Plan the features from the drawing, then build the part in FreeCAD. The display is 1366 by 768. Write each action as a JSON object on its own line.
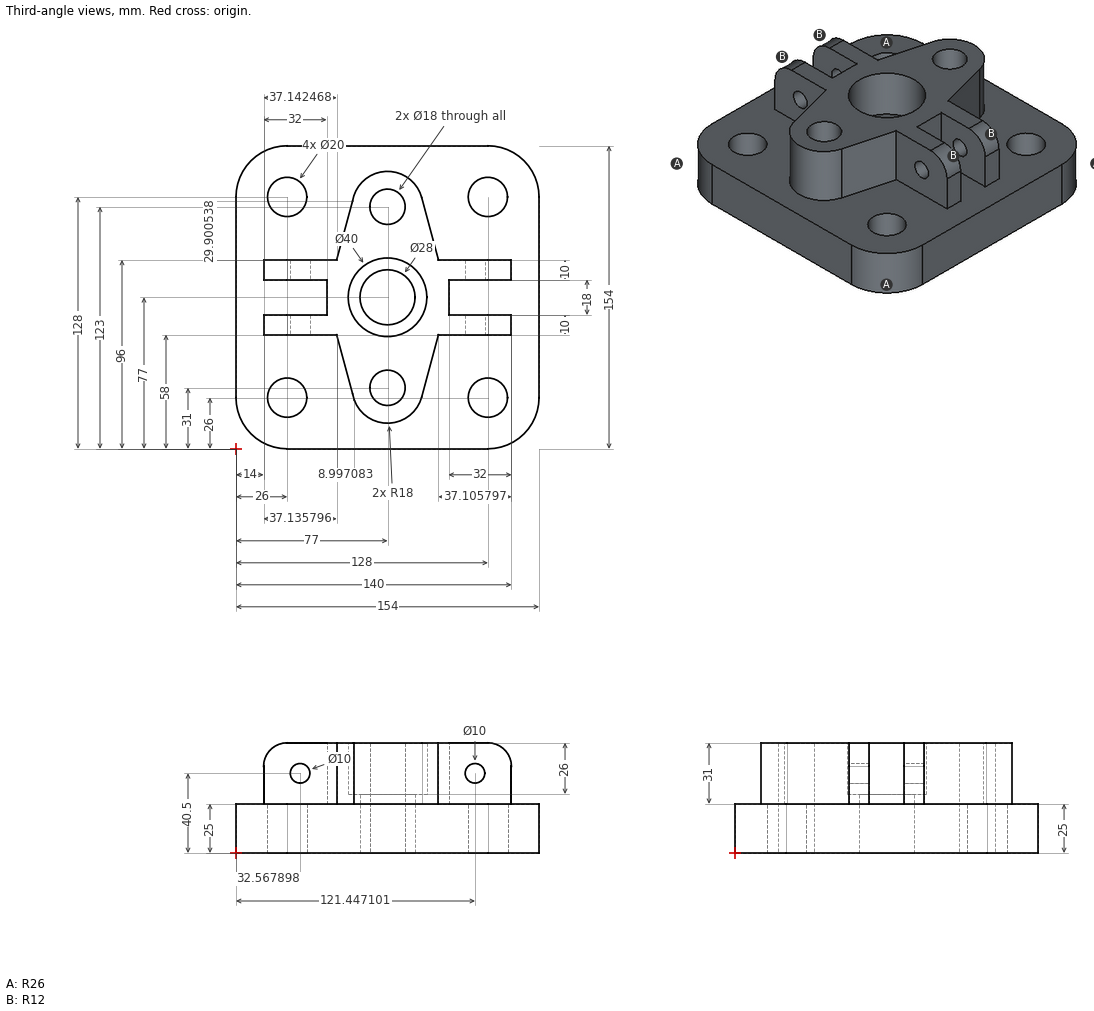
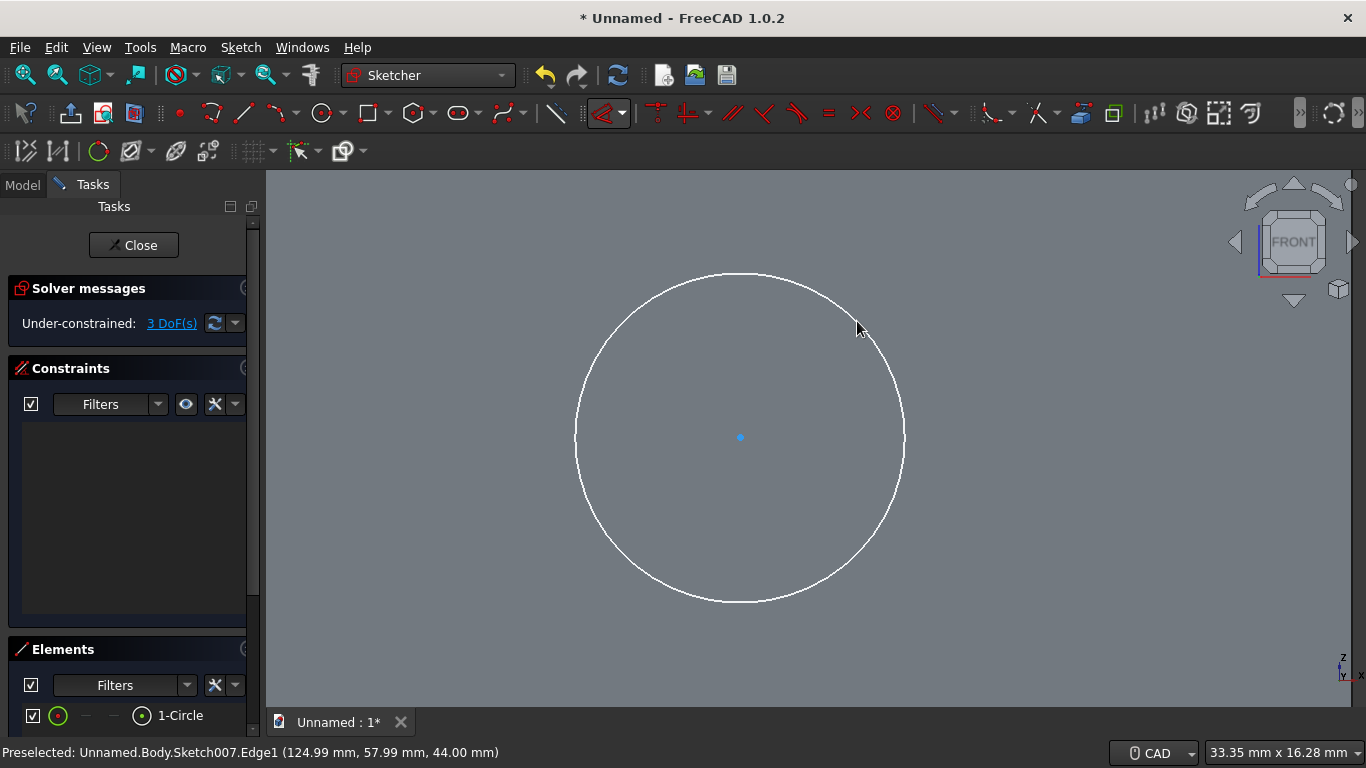
{"action": "left_click", "coordinate": [856, 321]}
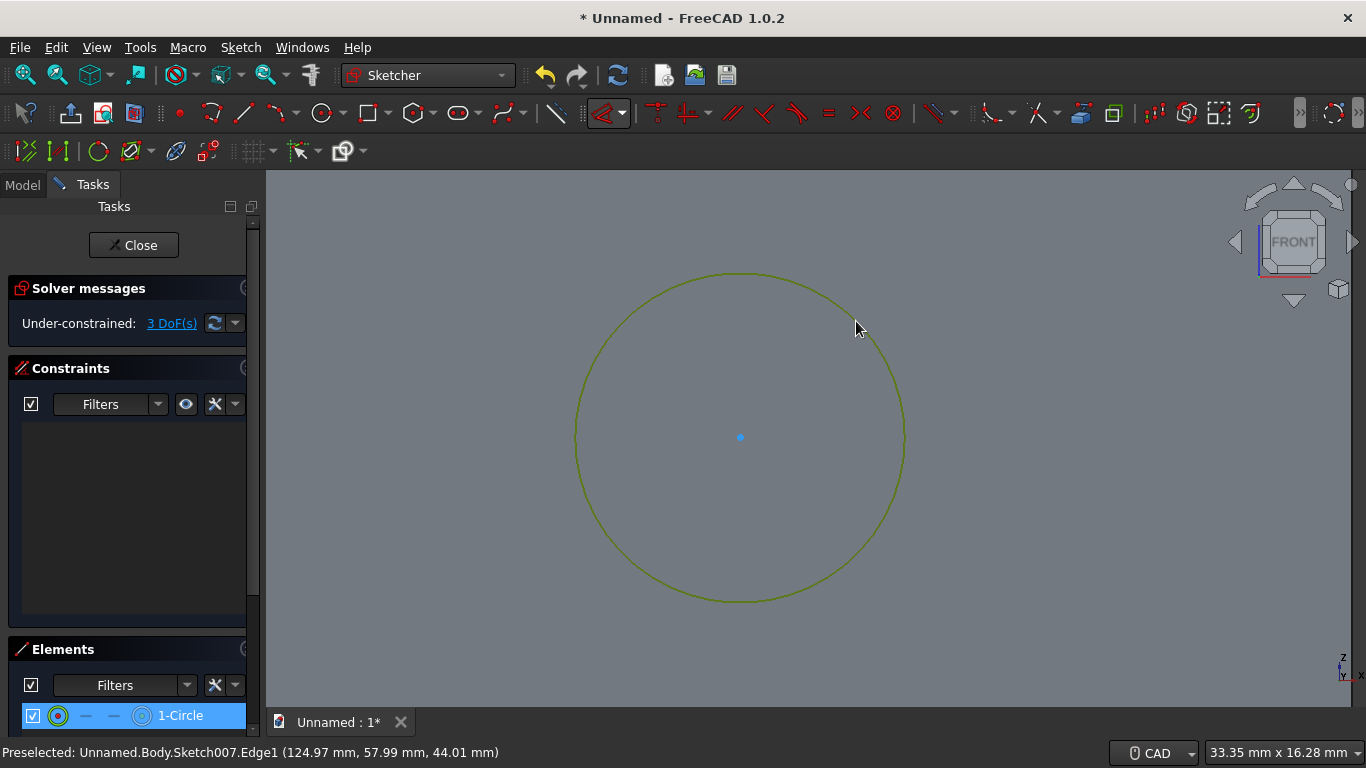
{"action": "left_click", "coordinate": [624, 114]}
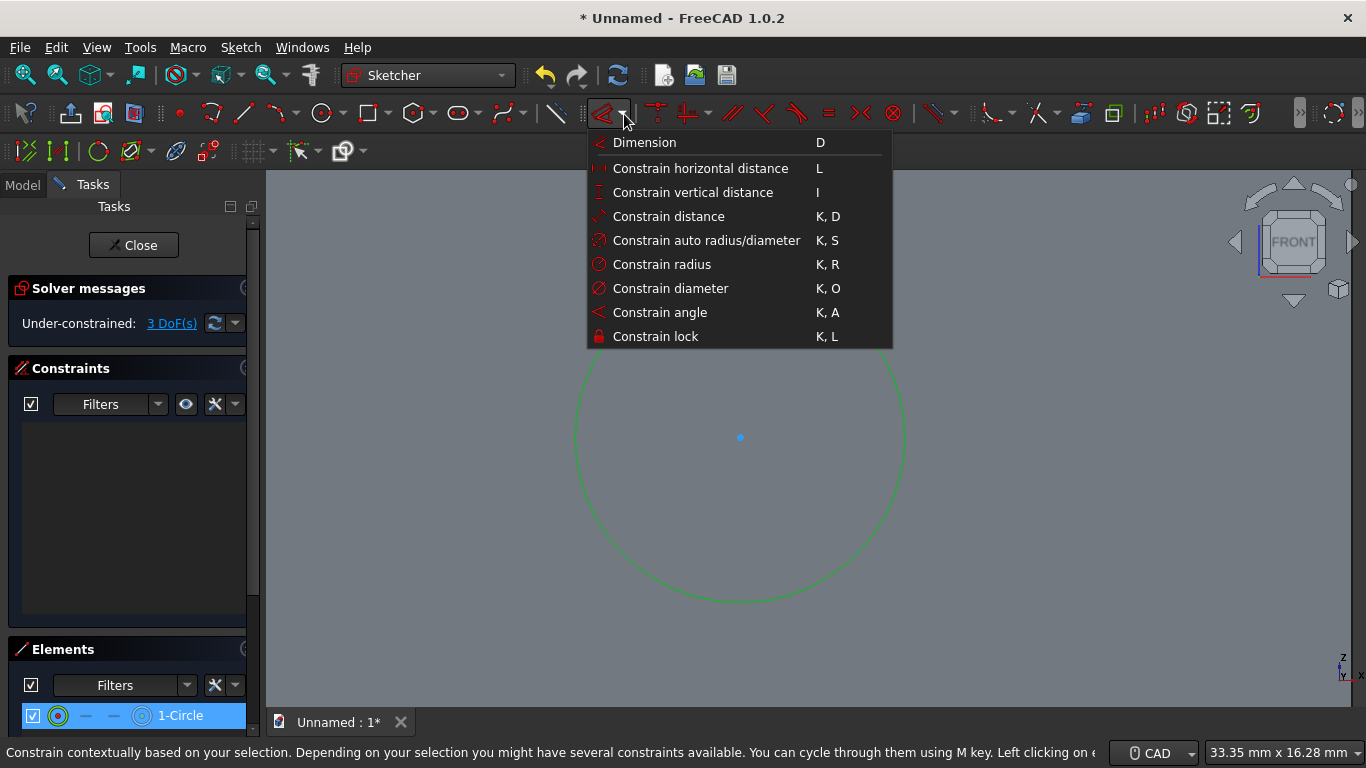
{"action": "left_click", "coordinate": [740, 288]}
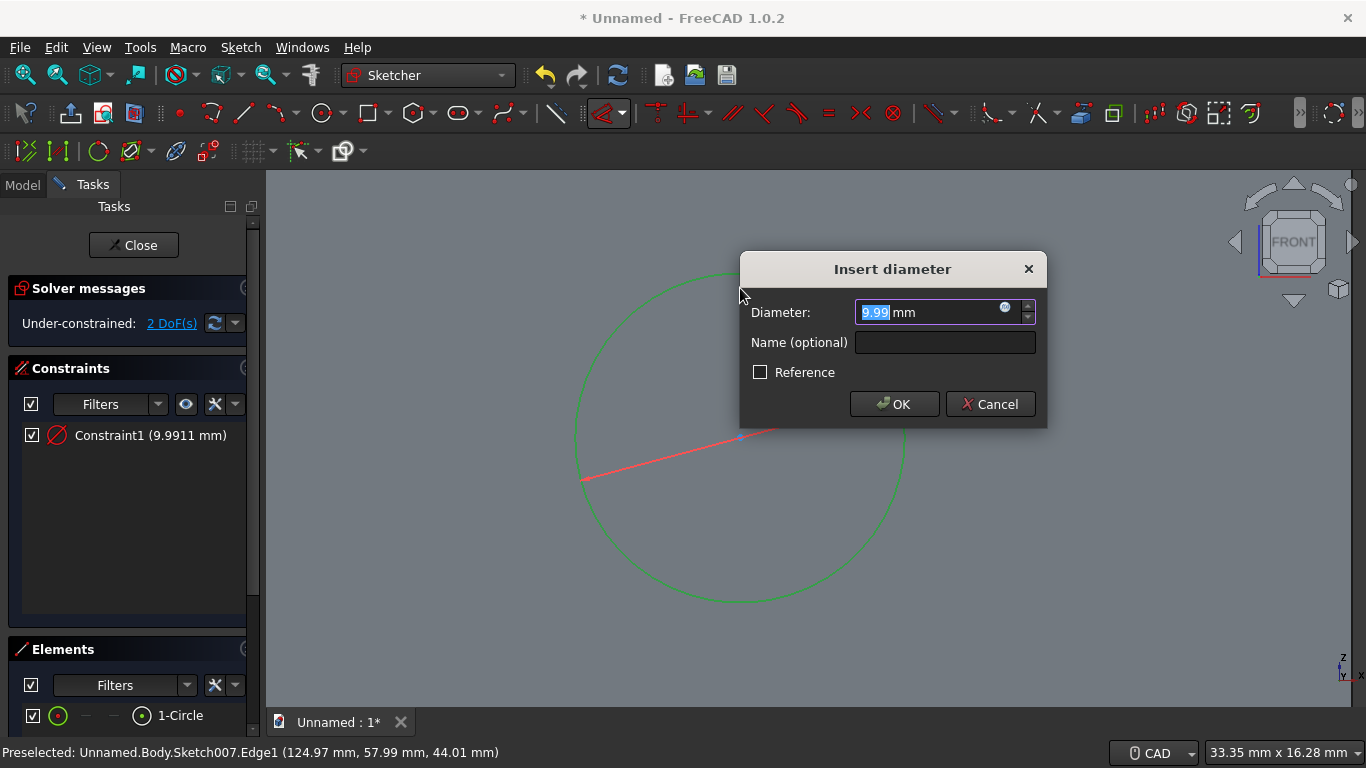
{"action": "type", "text": "10"}
{"action": "key", "text": "Return"}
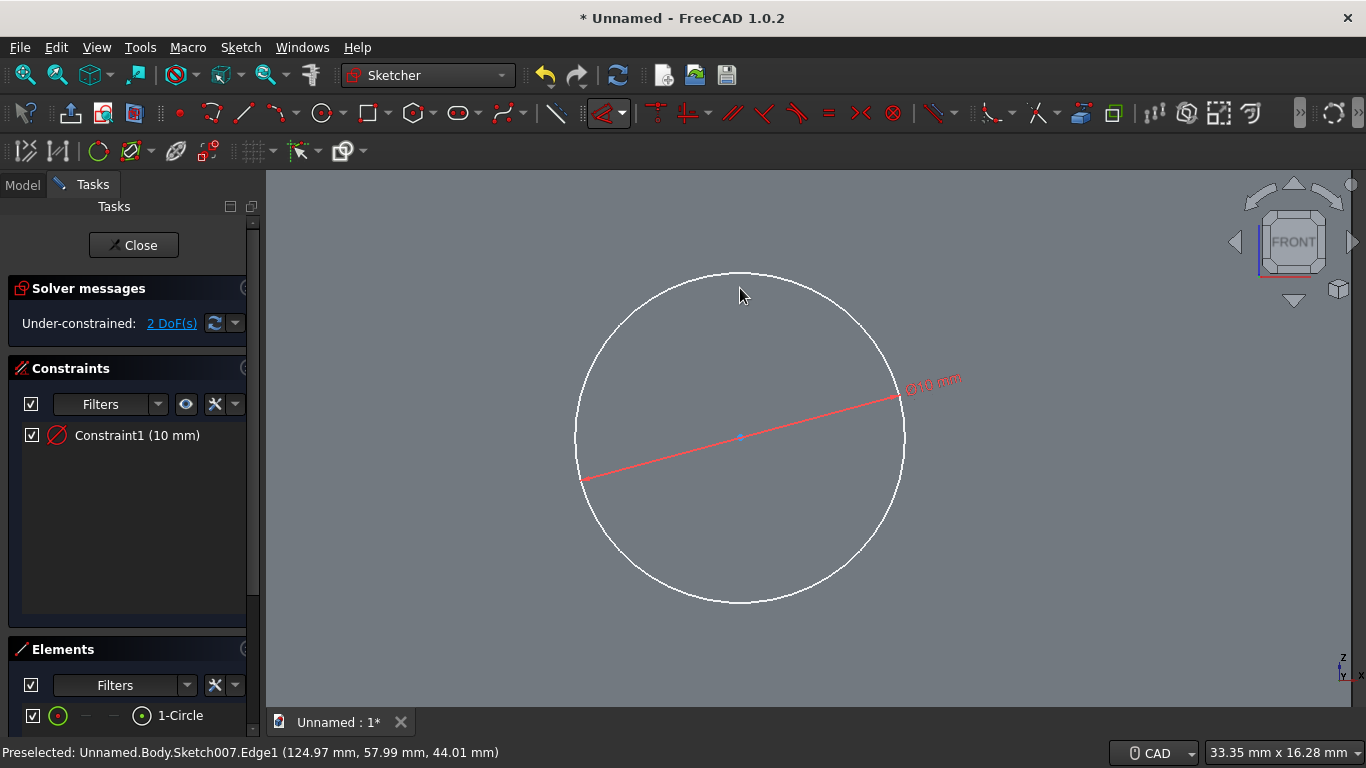
{"action": "left_click", "coordinate": [740, 438]}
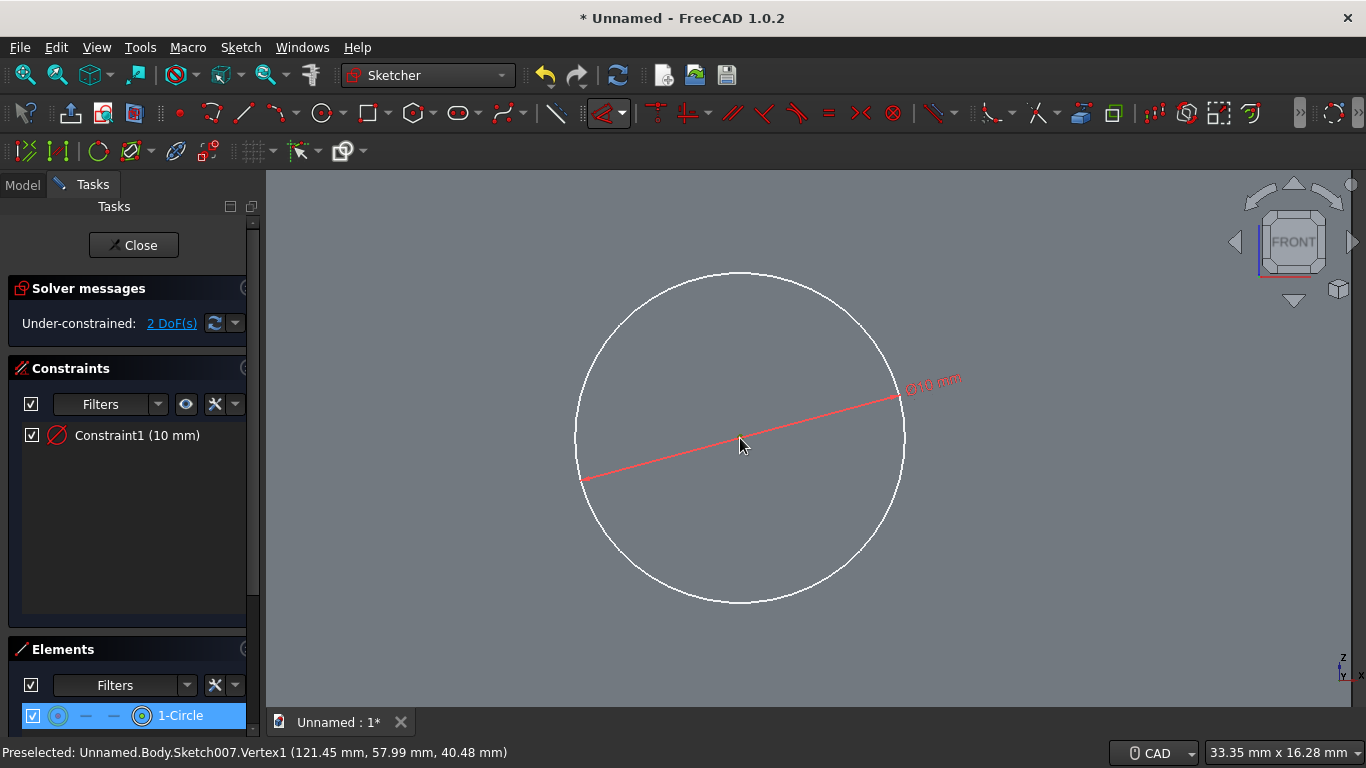
{"action": "left_click", "coordinate": [624, 114]}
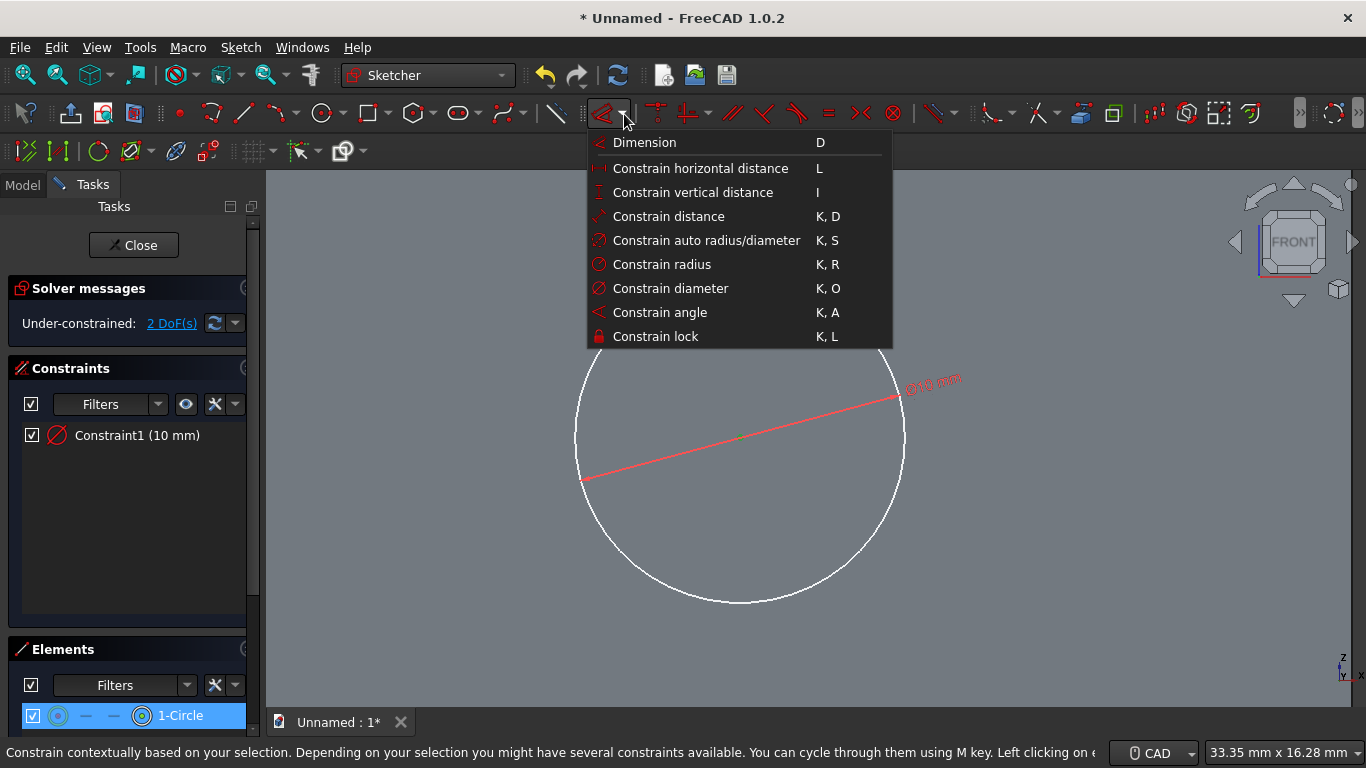
{"action": "left_click", "coordinate": [740, 192]}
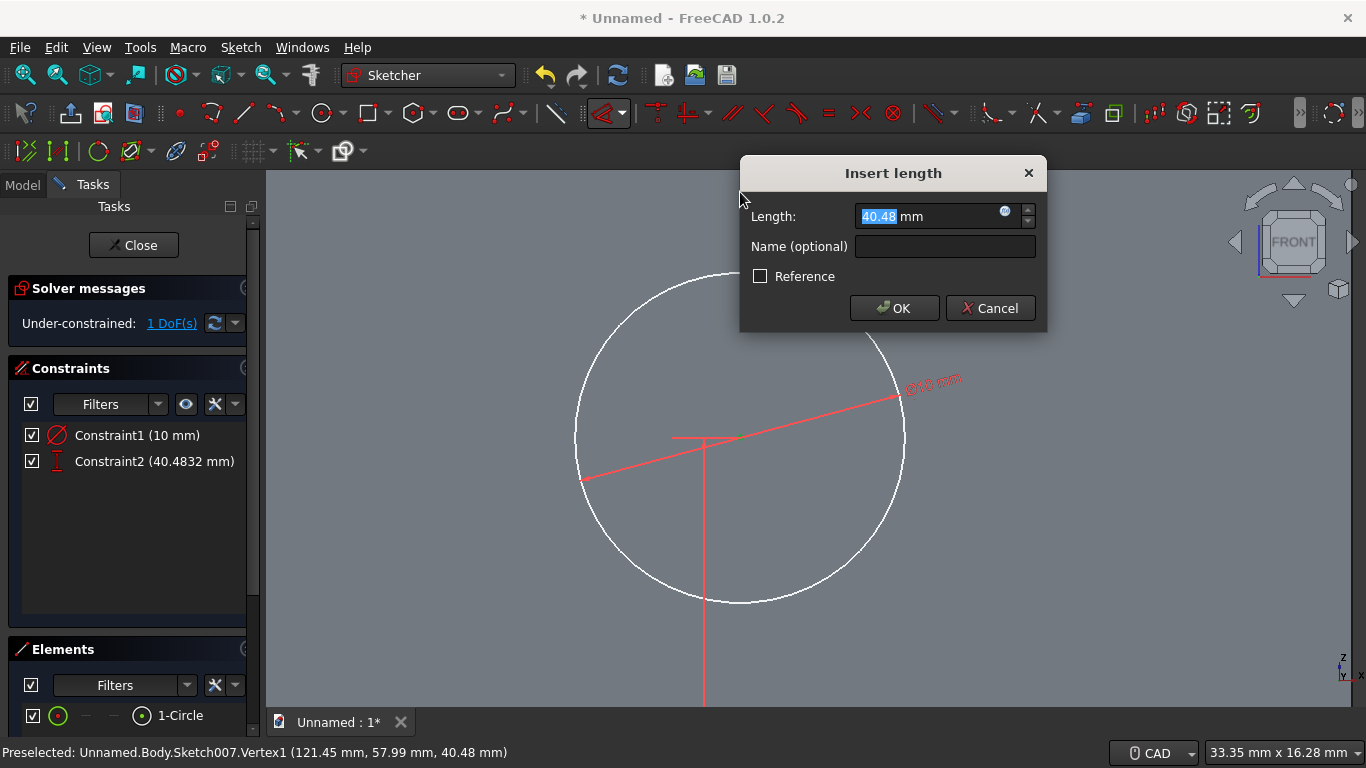
{"action": "type", "text": "40.5"}
{"action": "key", "text": "Return"}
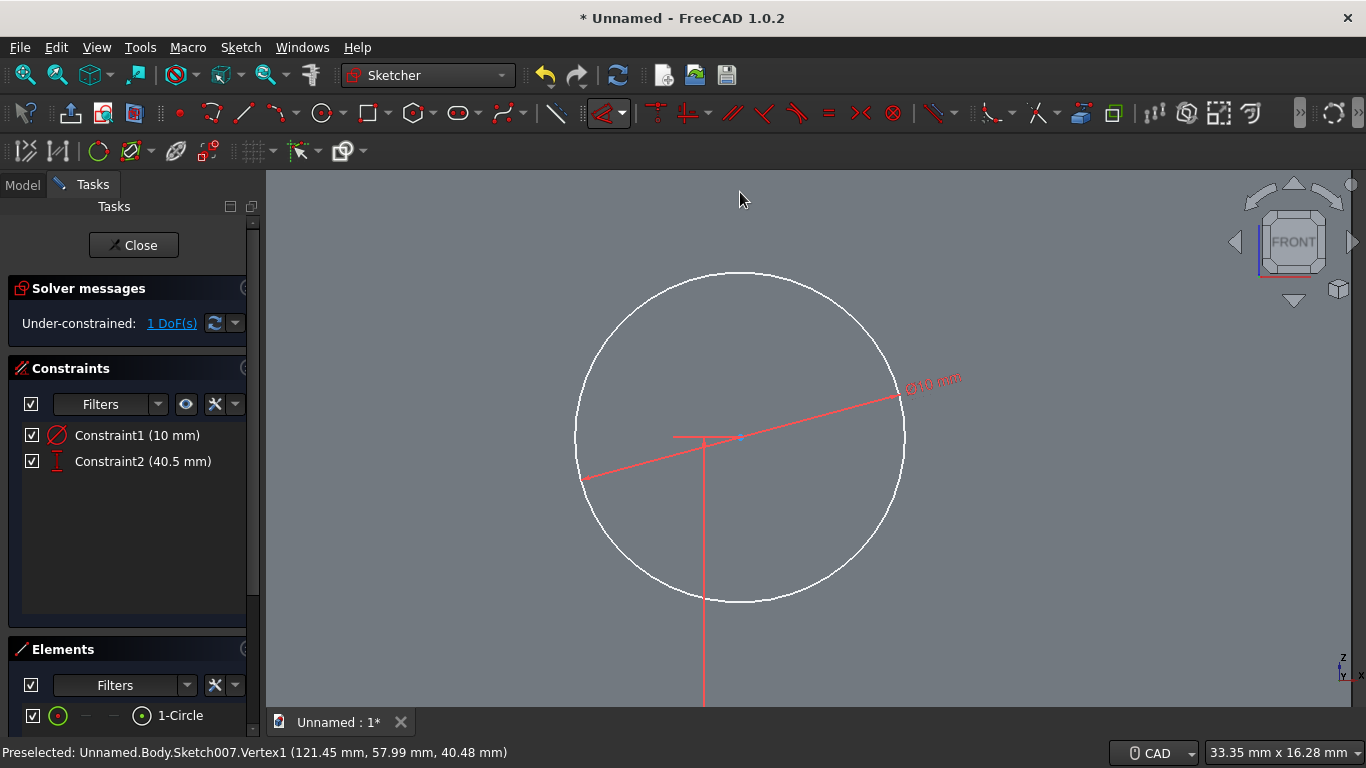
{"action": "left_click", "coordinate": [740, 437]}